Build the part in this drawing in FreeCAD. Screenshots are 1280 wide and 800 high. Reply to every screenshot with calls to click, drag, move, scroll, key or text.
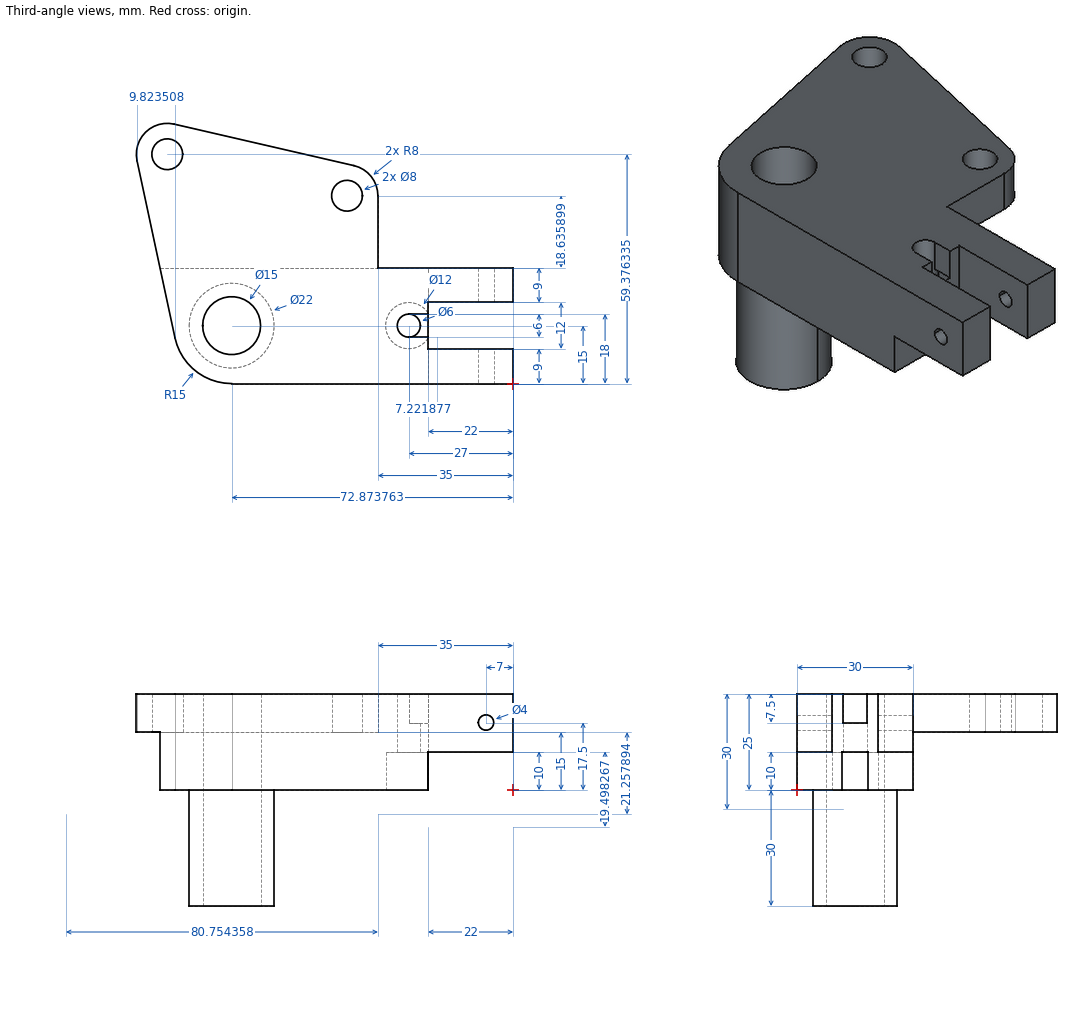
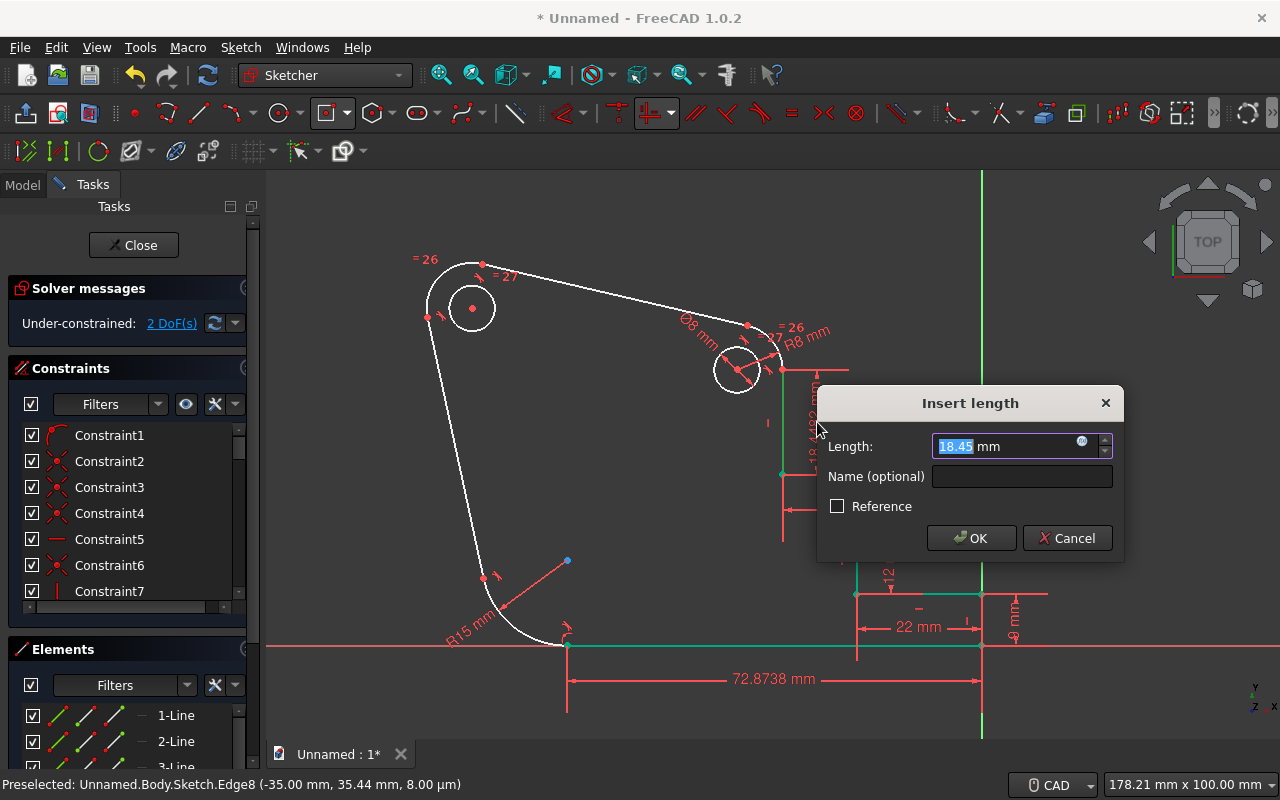
text(18.635899)
key(Return)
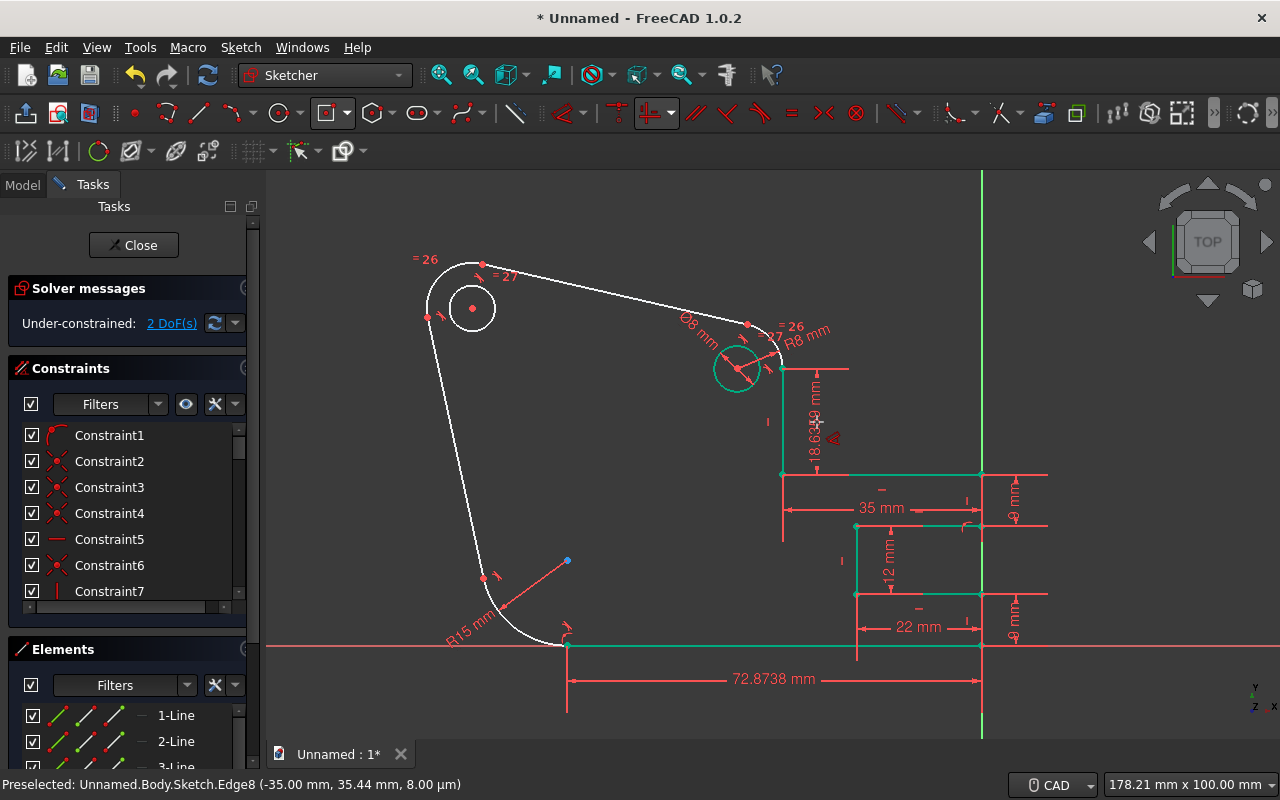
click(445, 396)
click(436, 260)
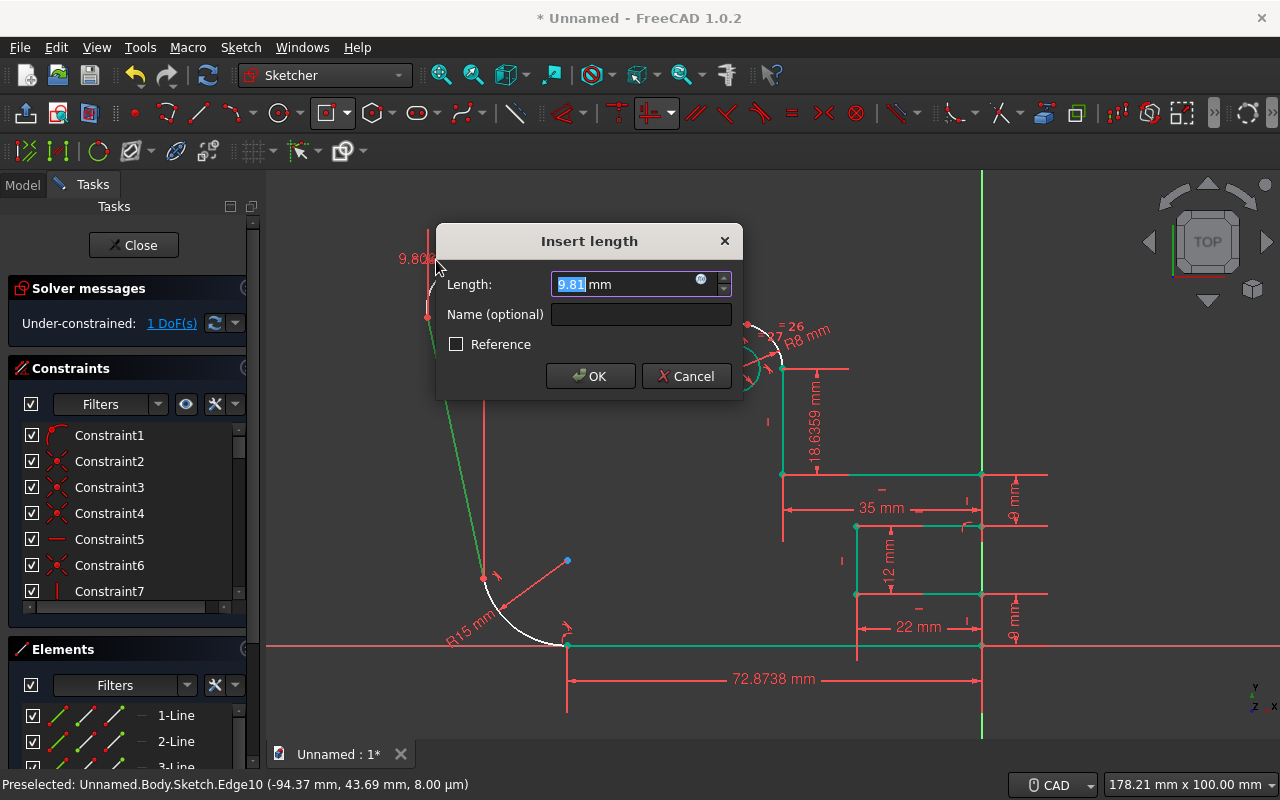
text(9.823508)
key(Return)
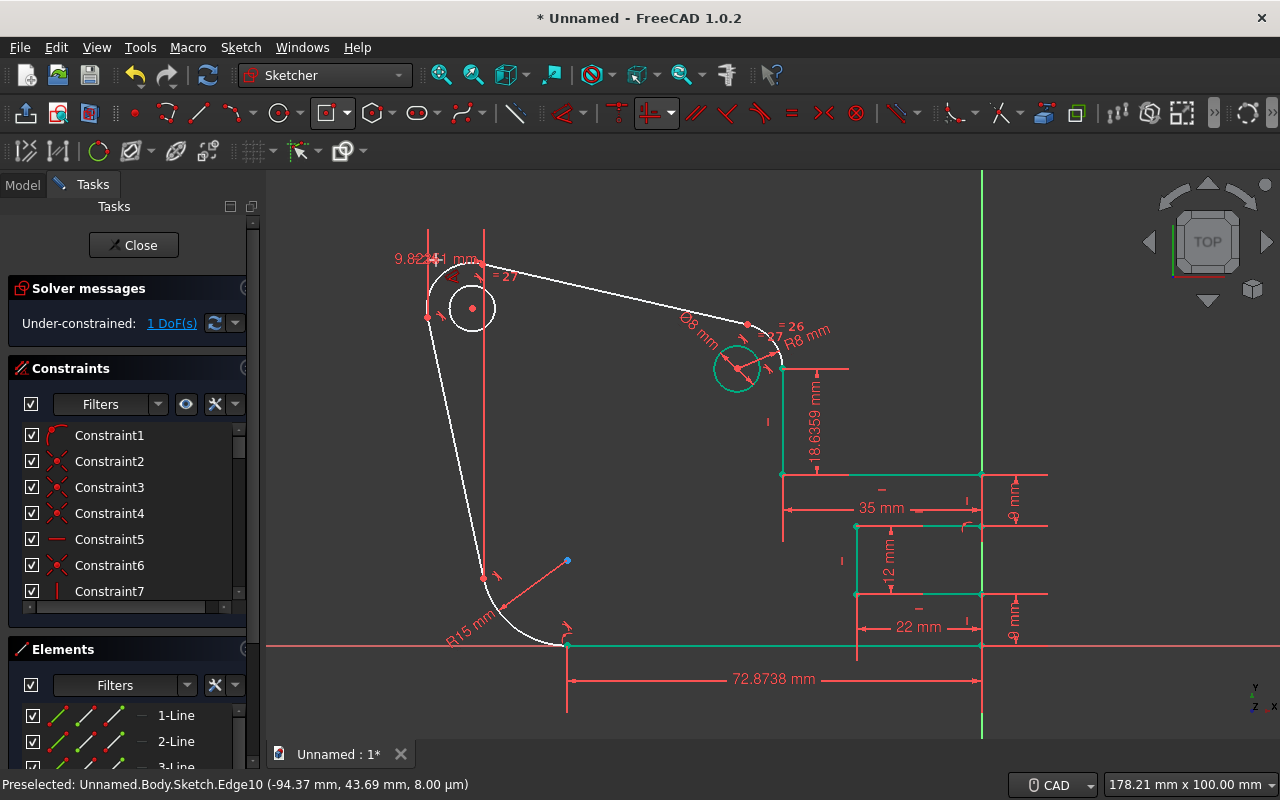
click(472, 308)
click(1016, 477)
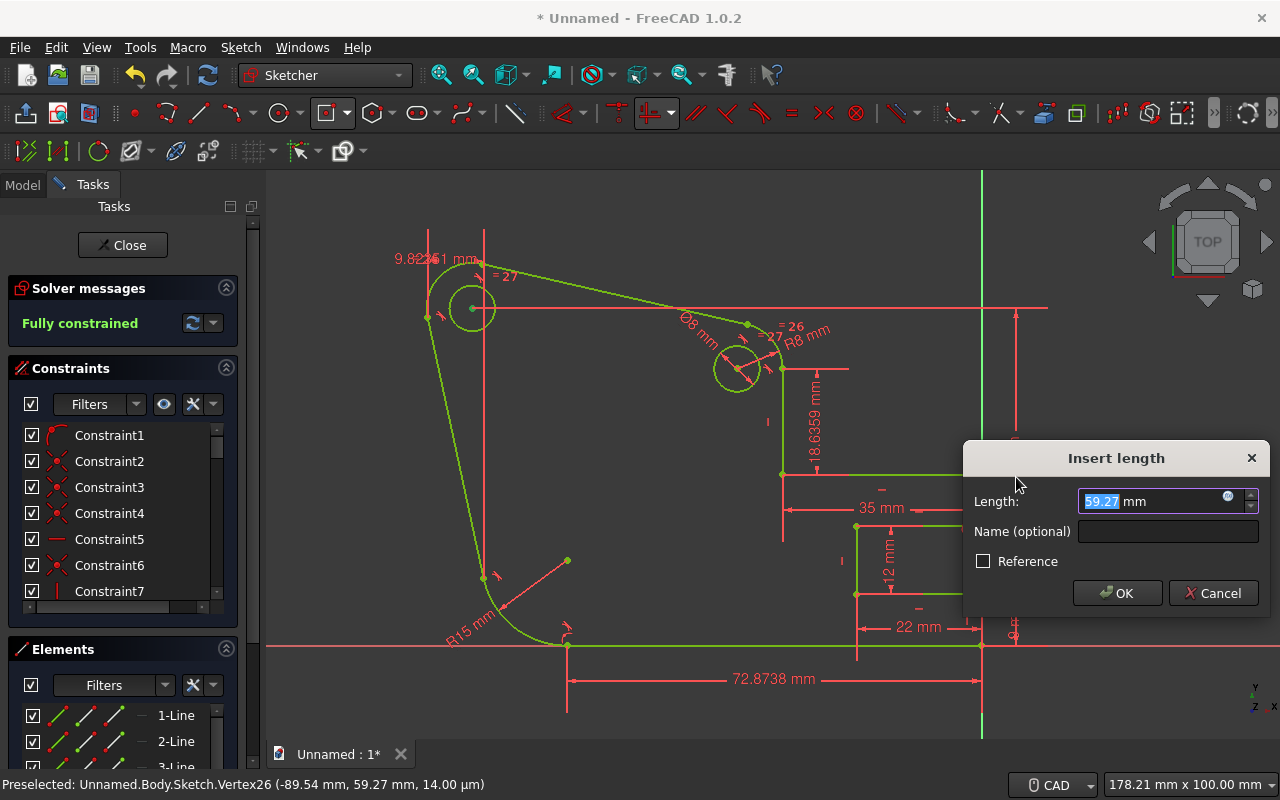
text(59.376335)
key(Return)
key(Escape)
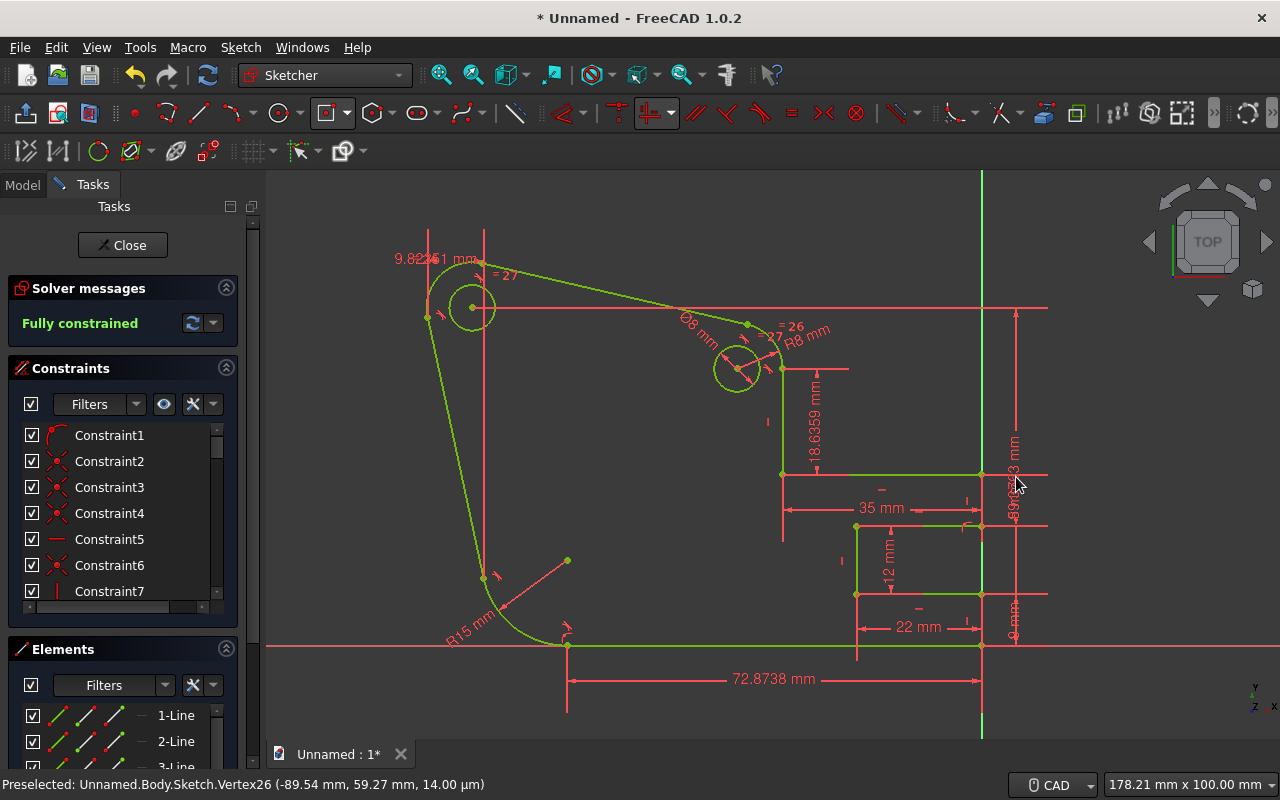
click(123, 245)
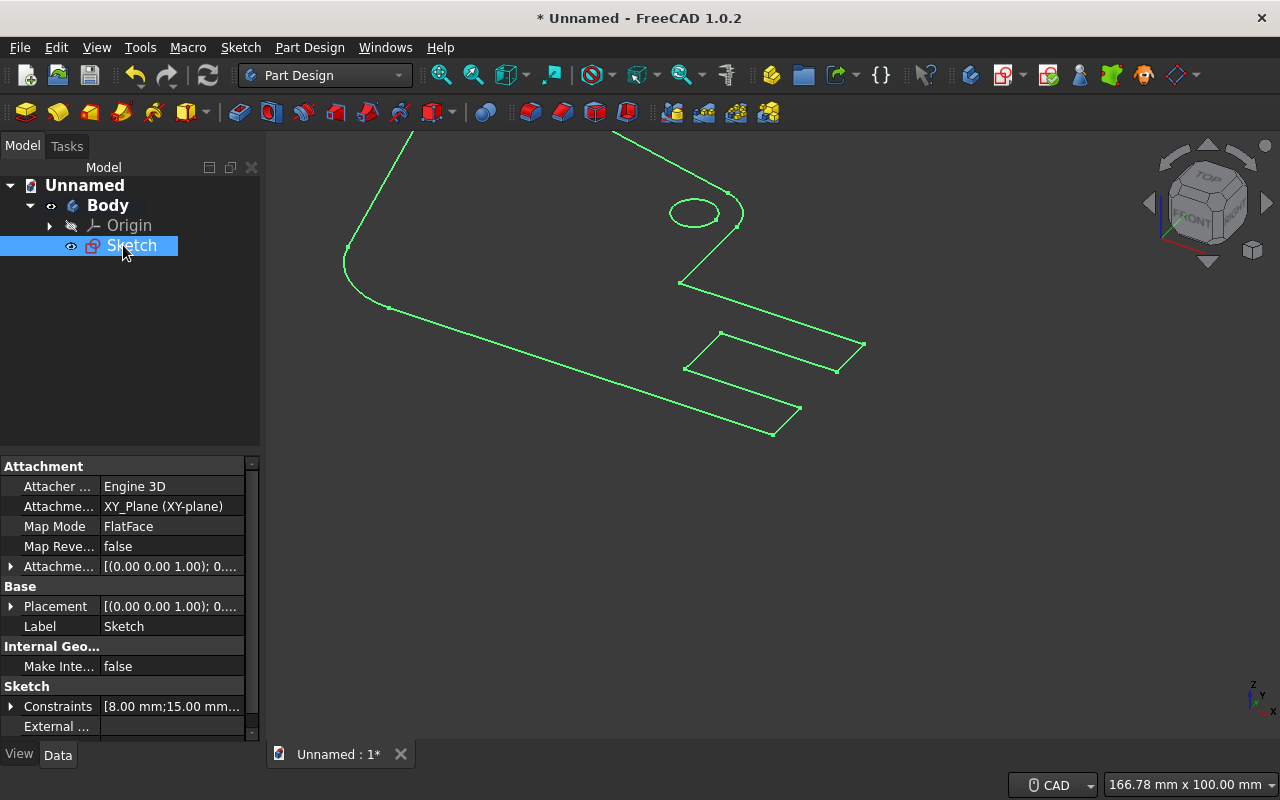
click(26, 112)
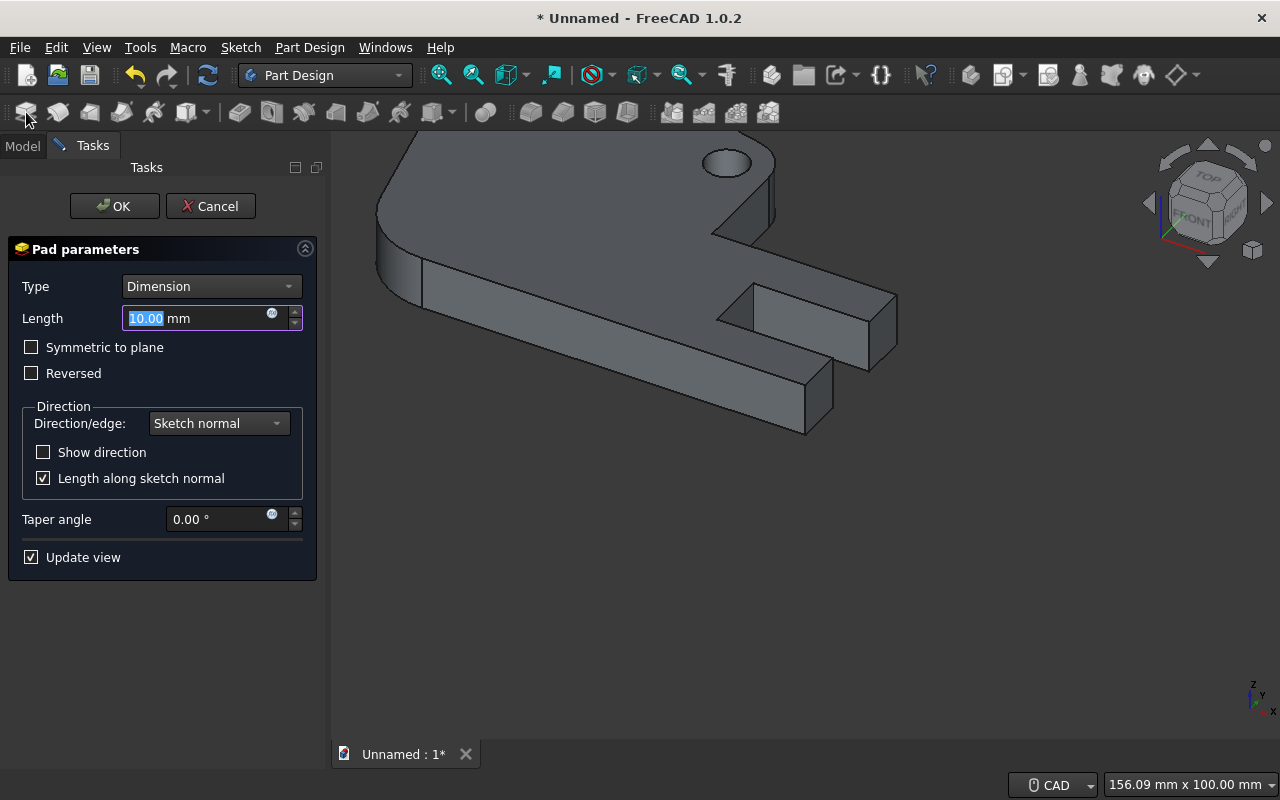
text(25)
key(Tab)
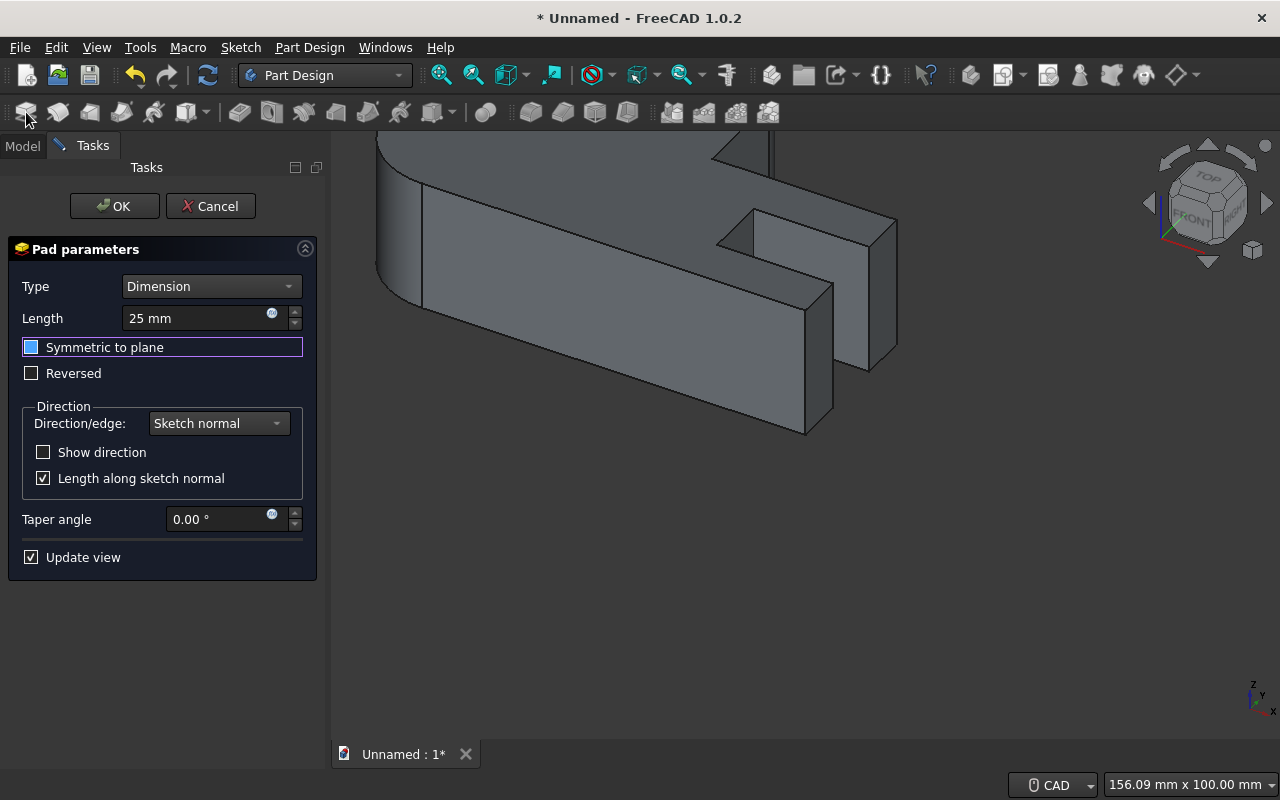
click(115, 206)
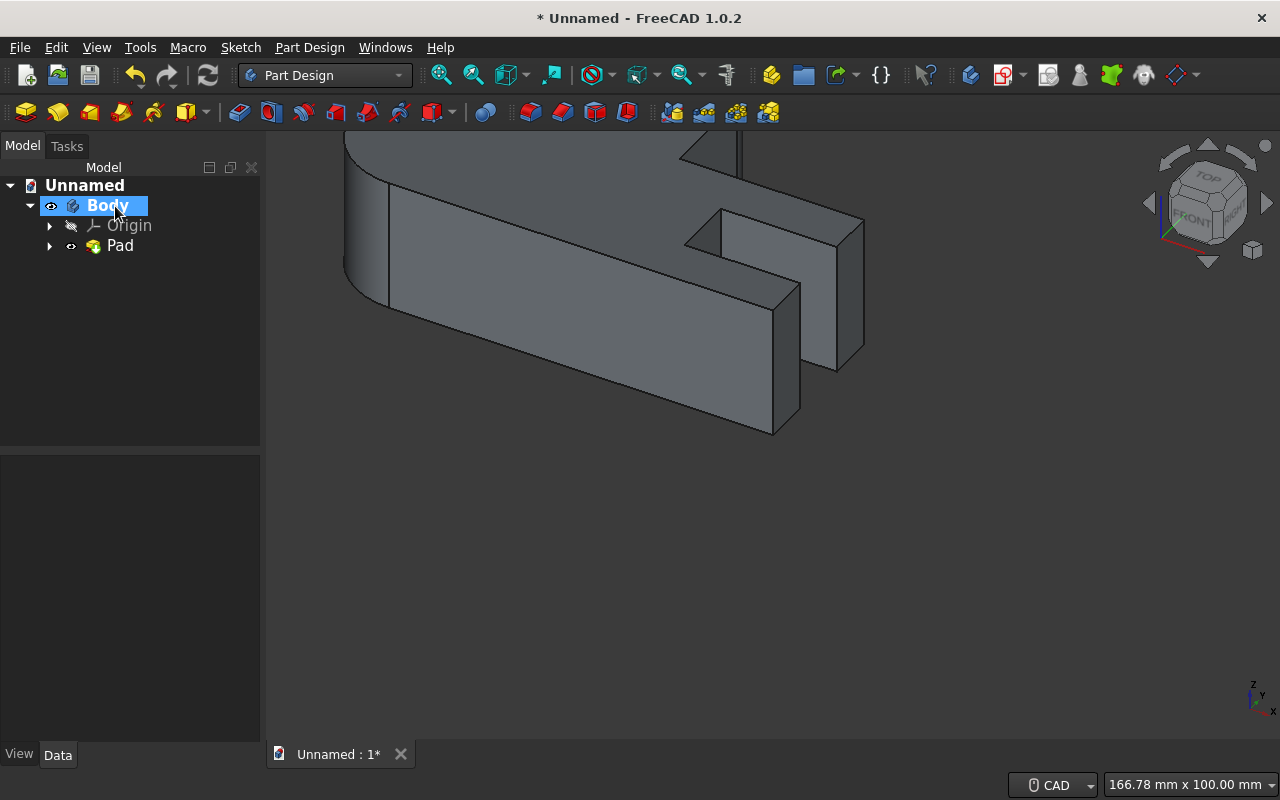
key(v)
key(f)